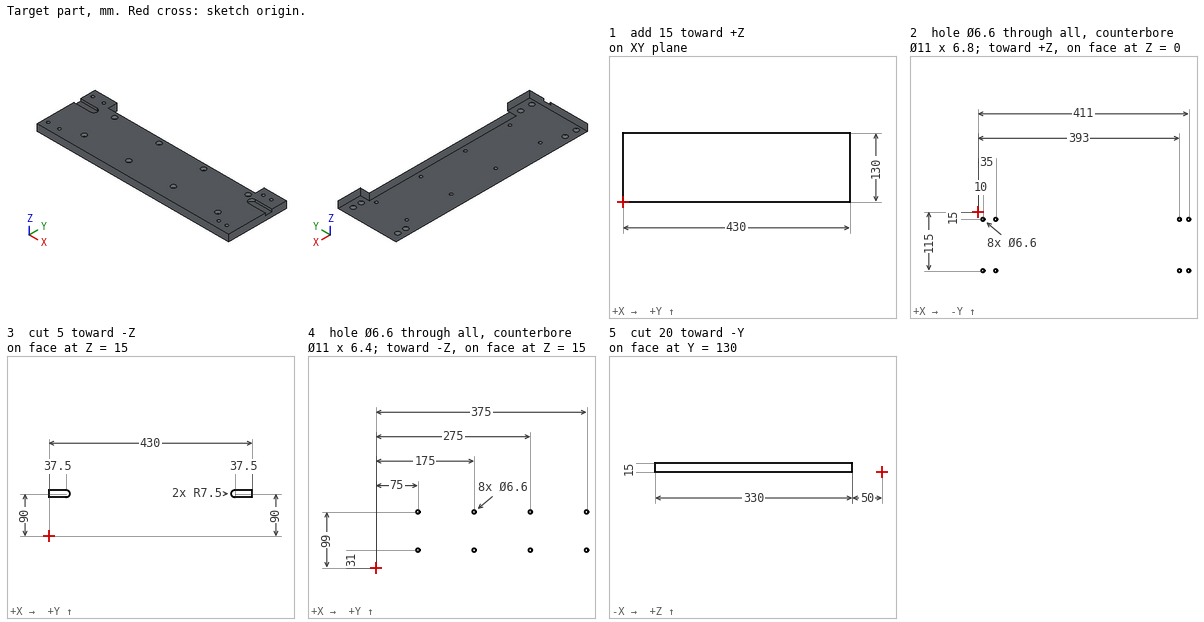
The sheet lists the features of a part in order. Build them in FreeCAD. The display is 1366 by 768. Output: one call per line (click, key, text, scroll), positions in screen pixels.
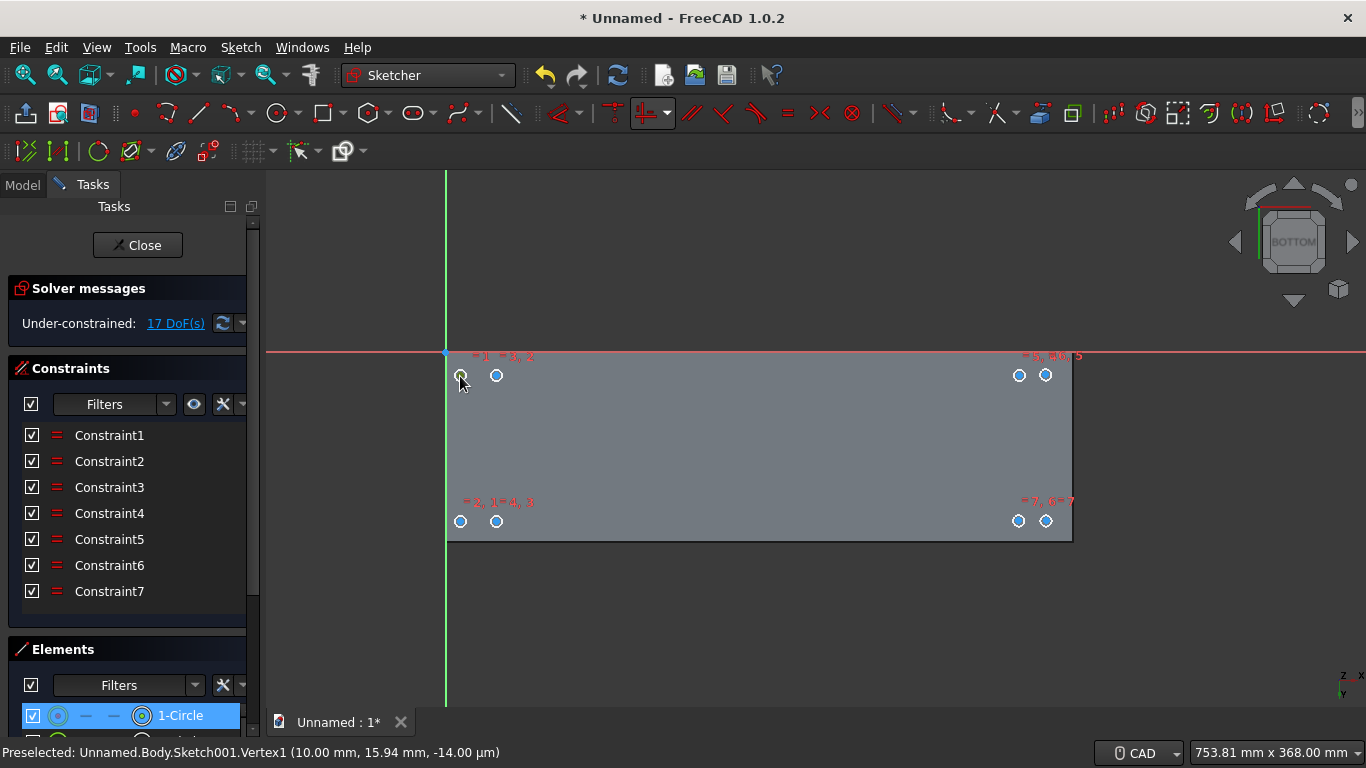
click(460, 522)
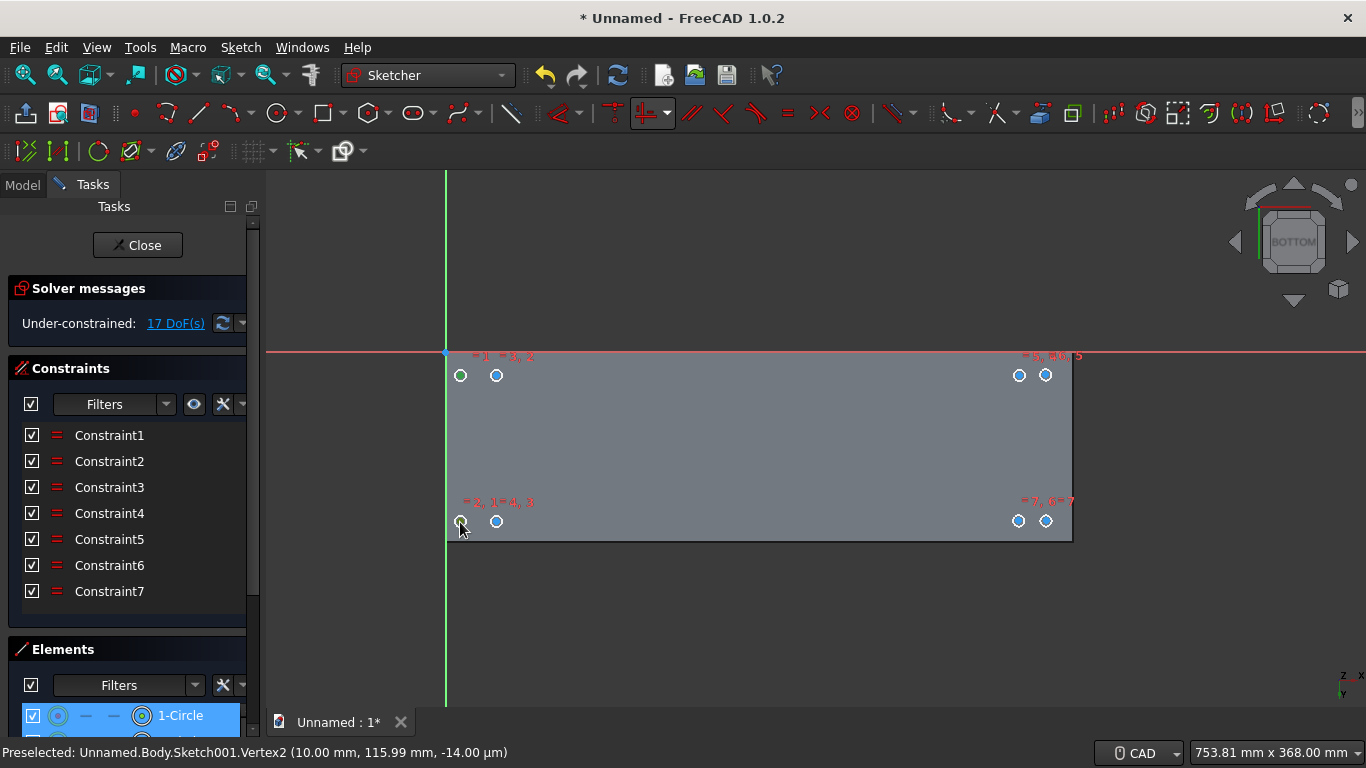
click(670, 114)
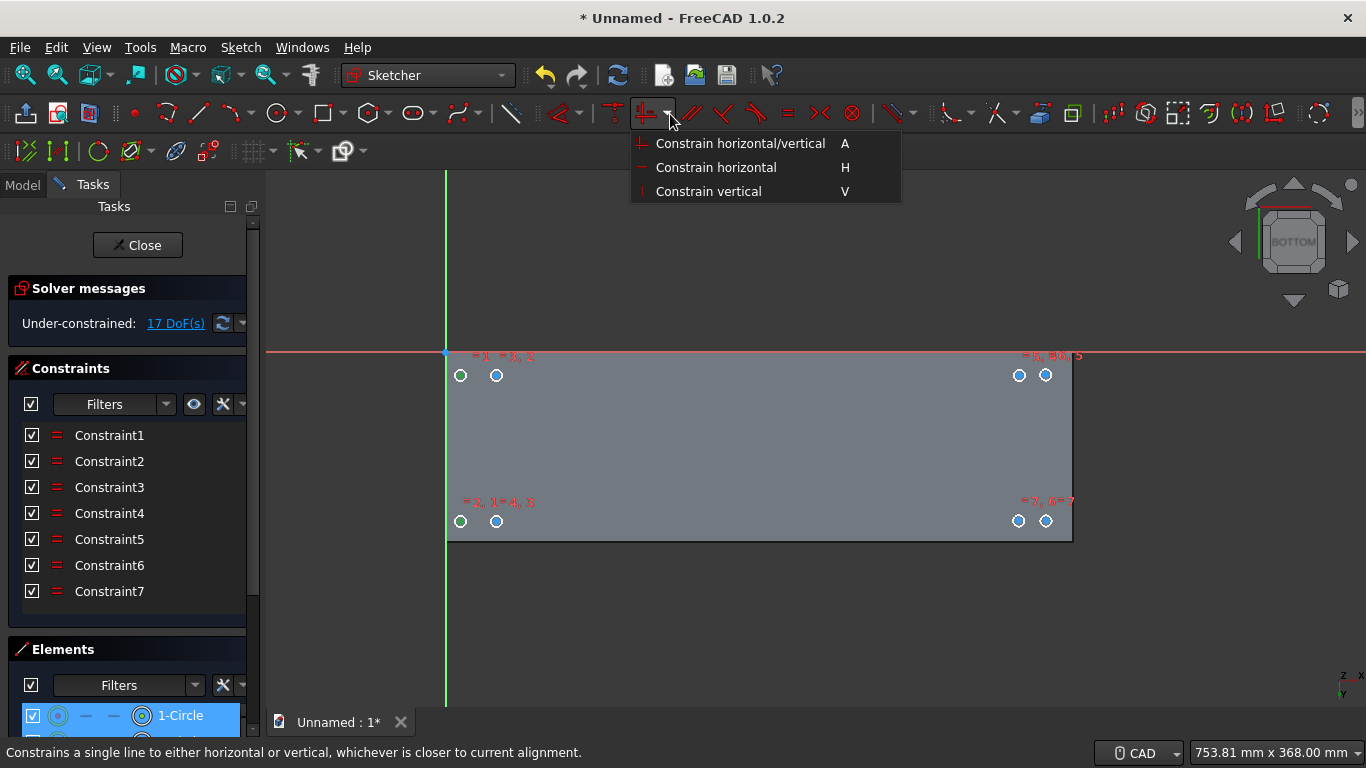
click(766, 191)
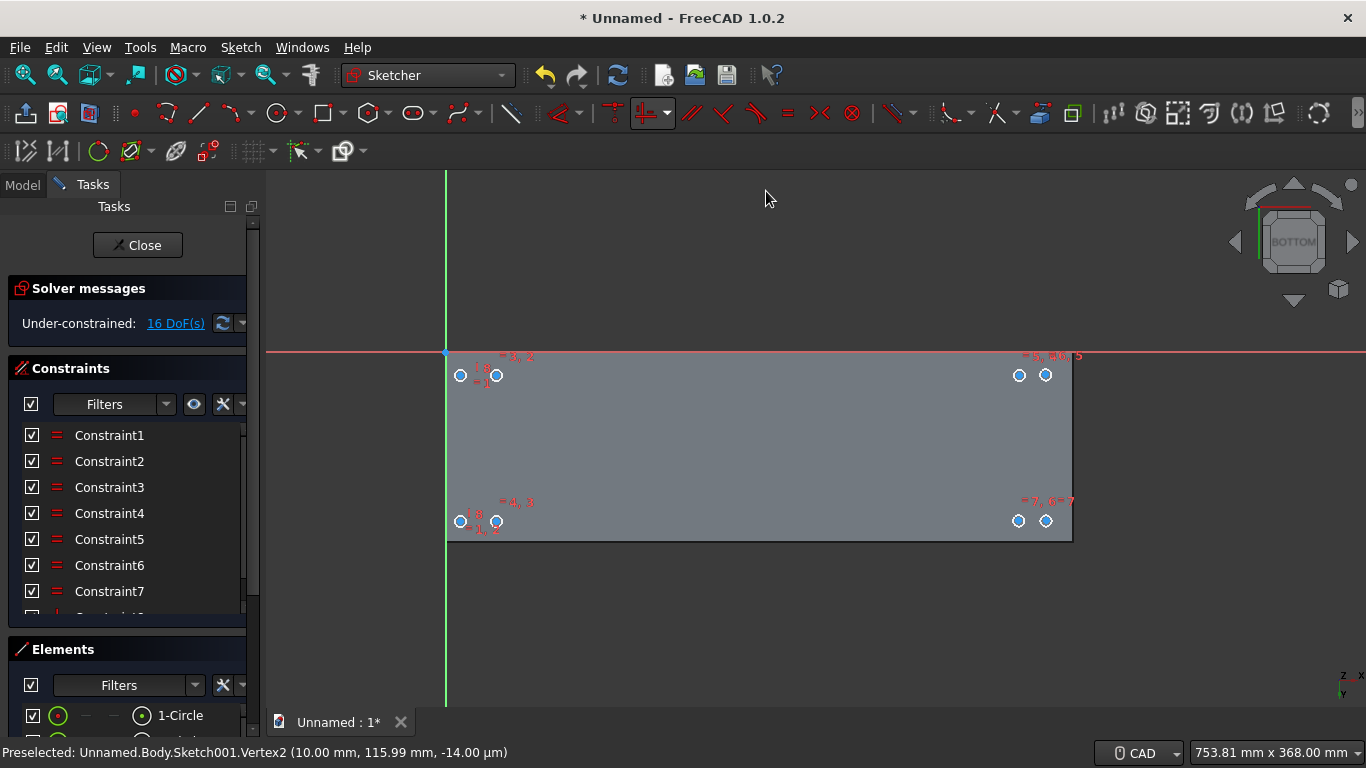
click(460, 376)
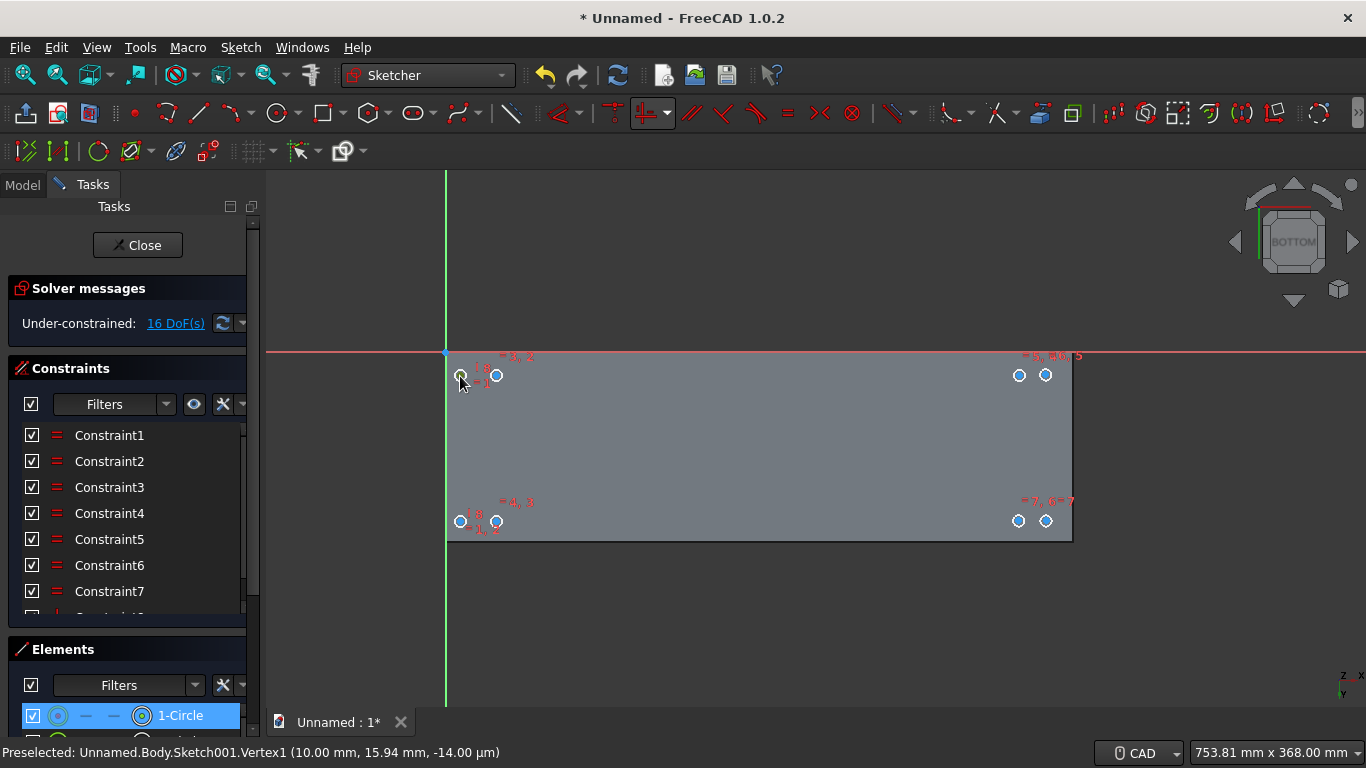
click(496, 376)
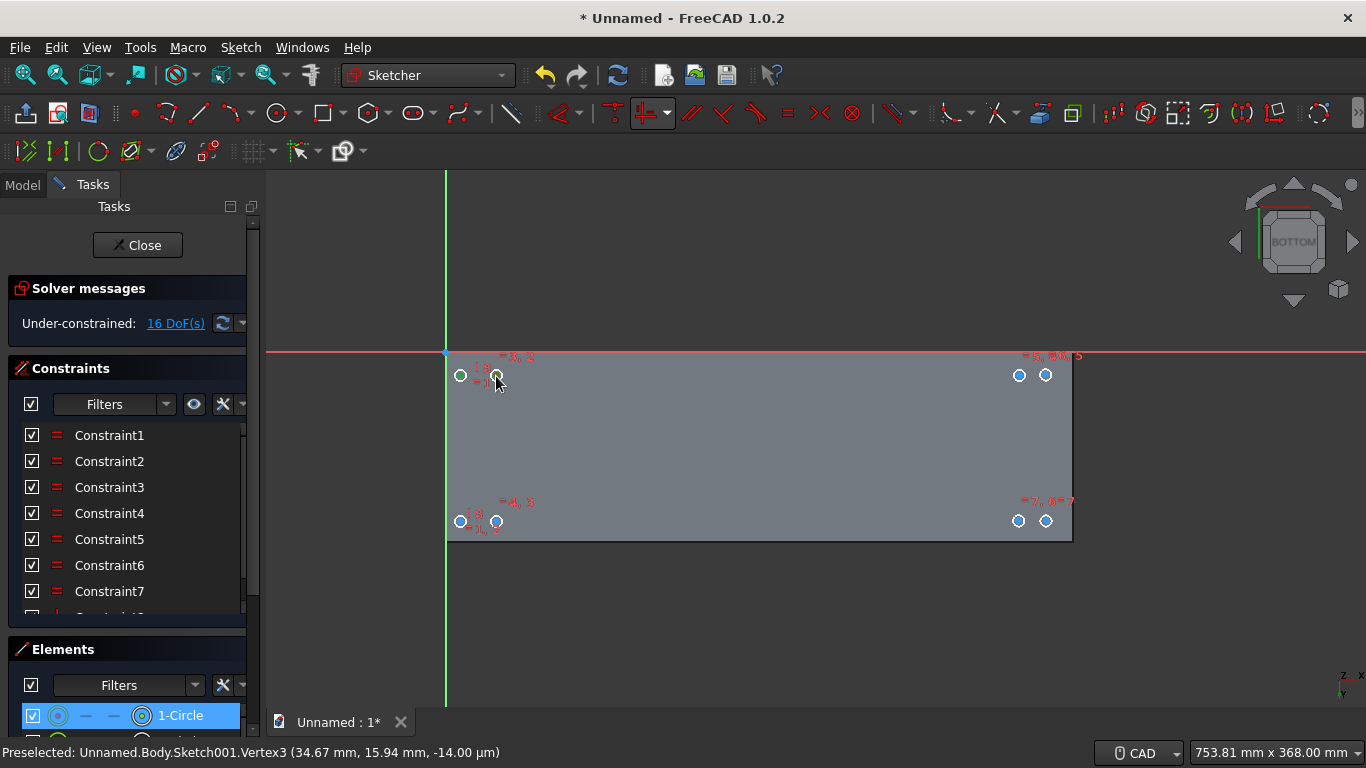
key(h)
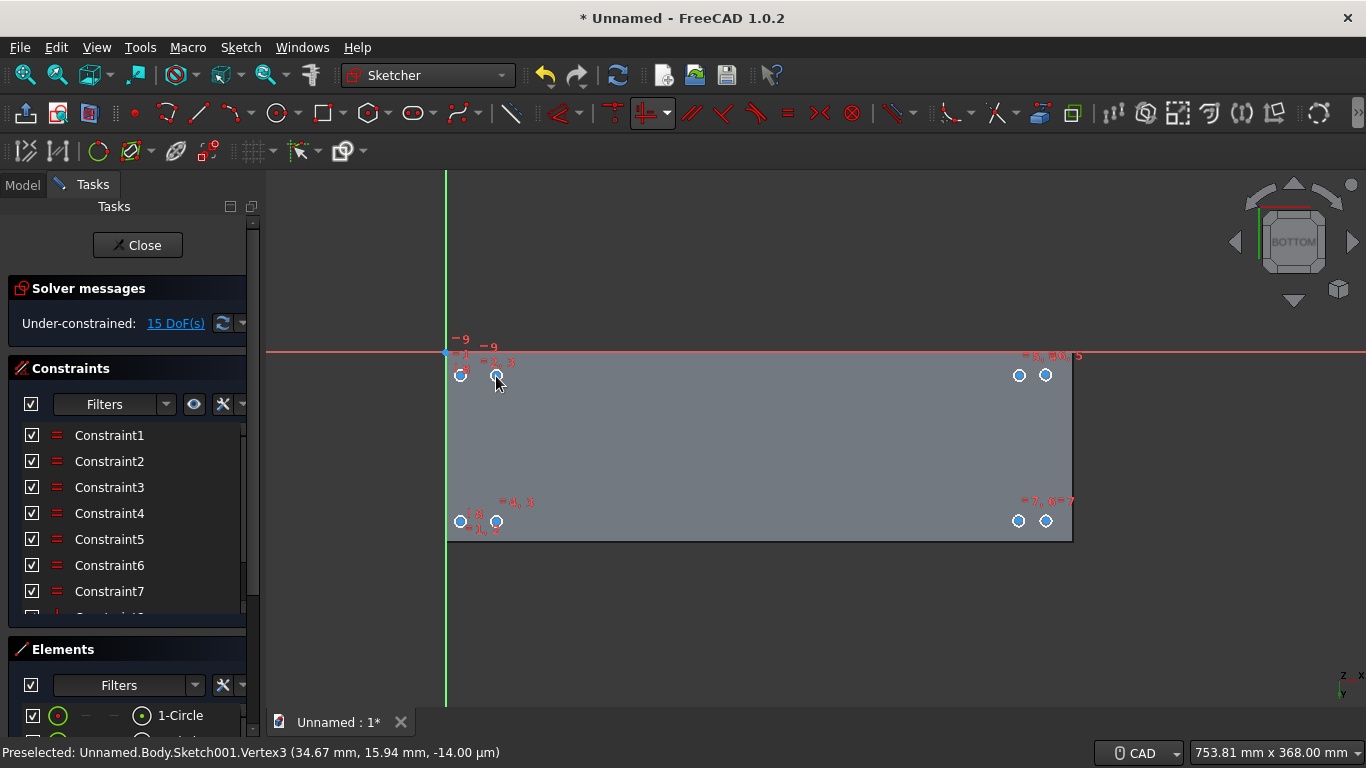
click(496, 376)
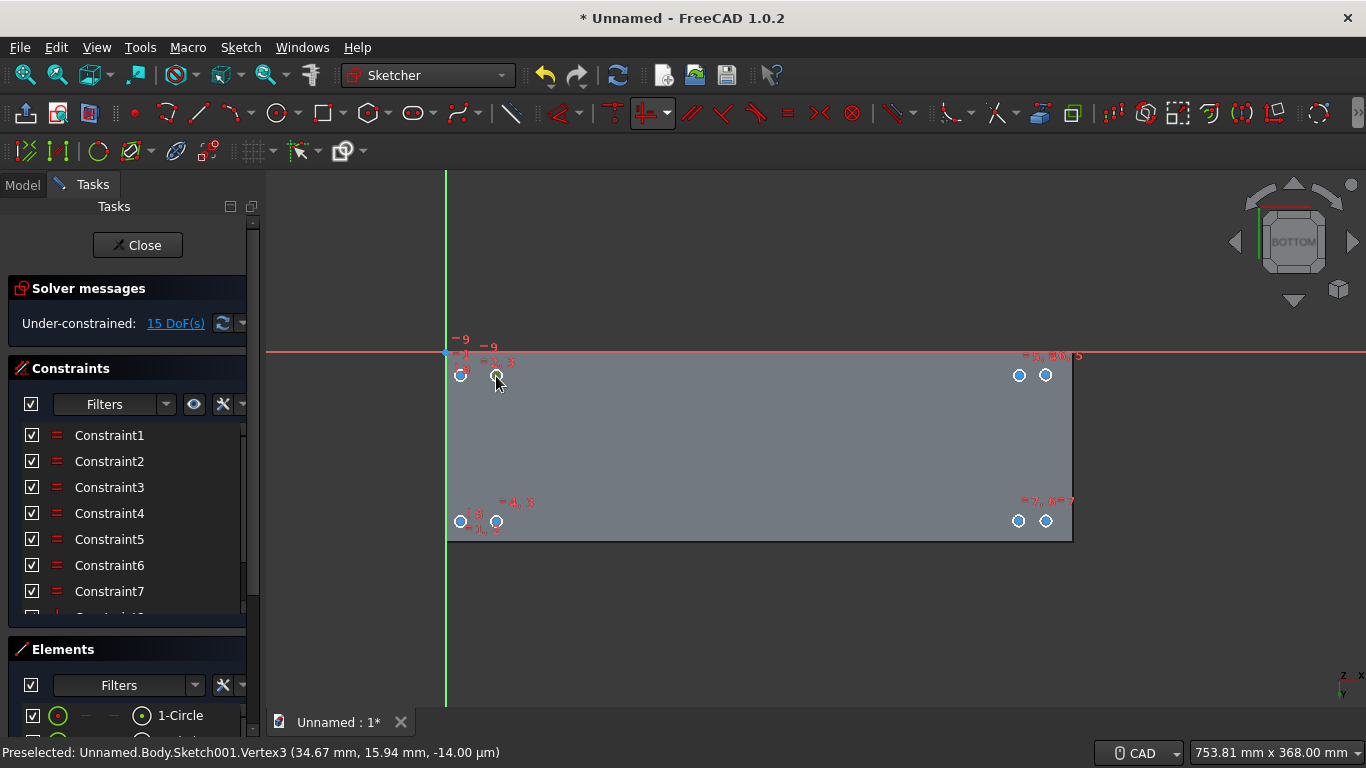
scroll(496, 522, up, 4)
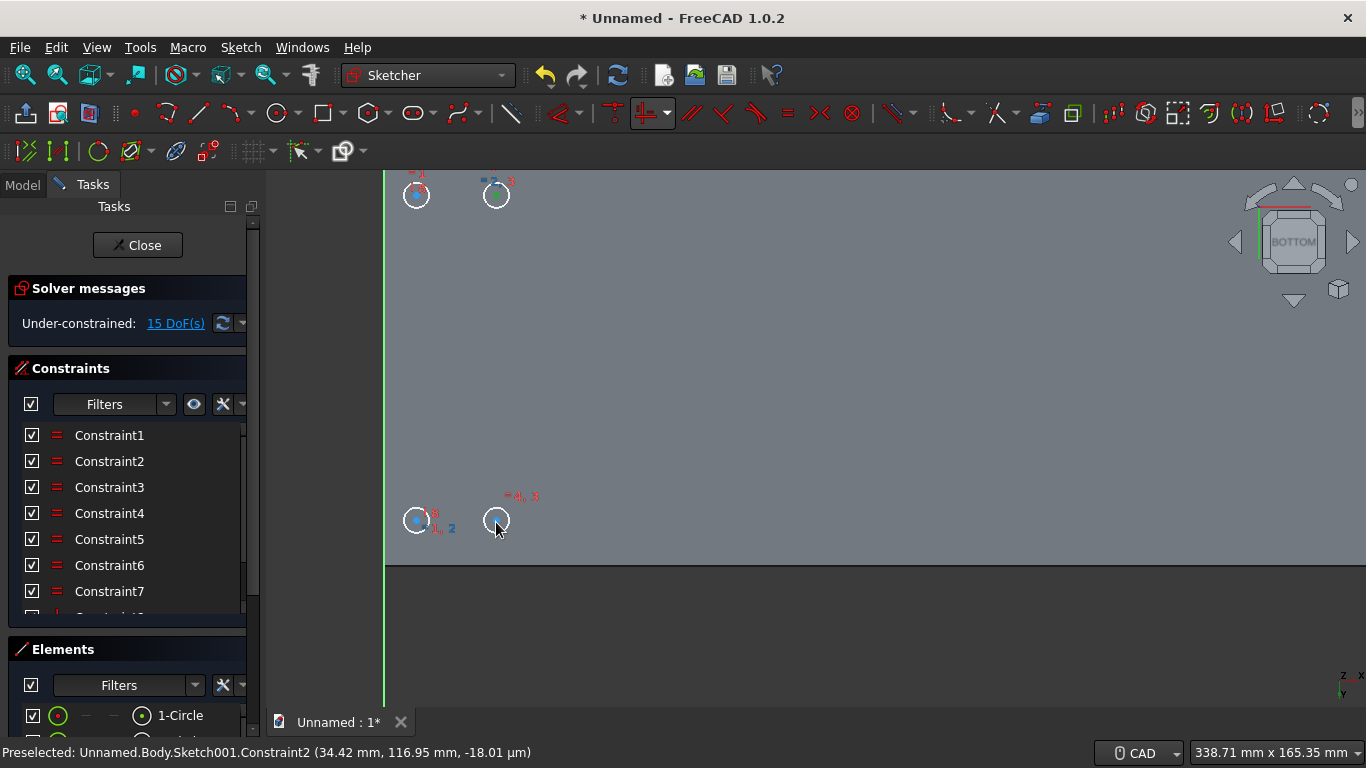
click(497, 520)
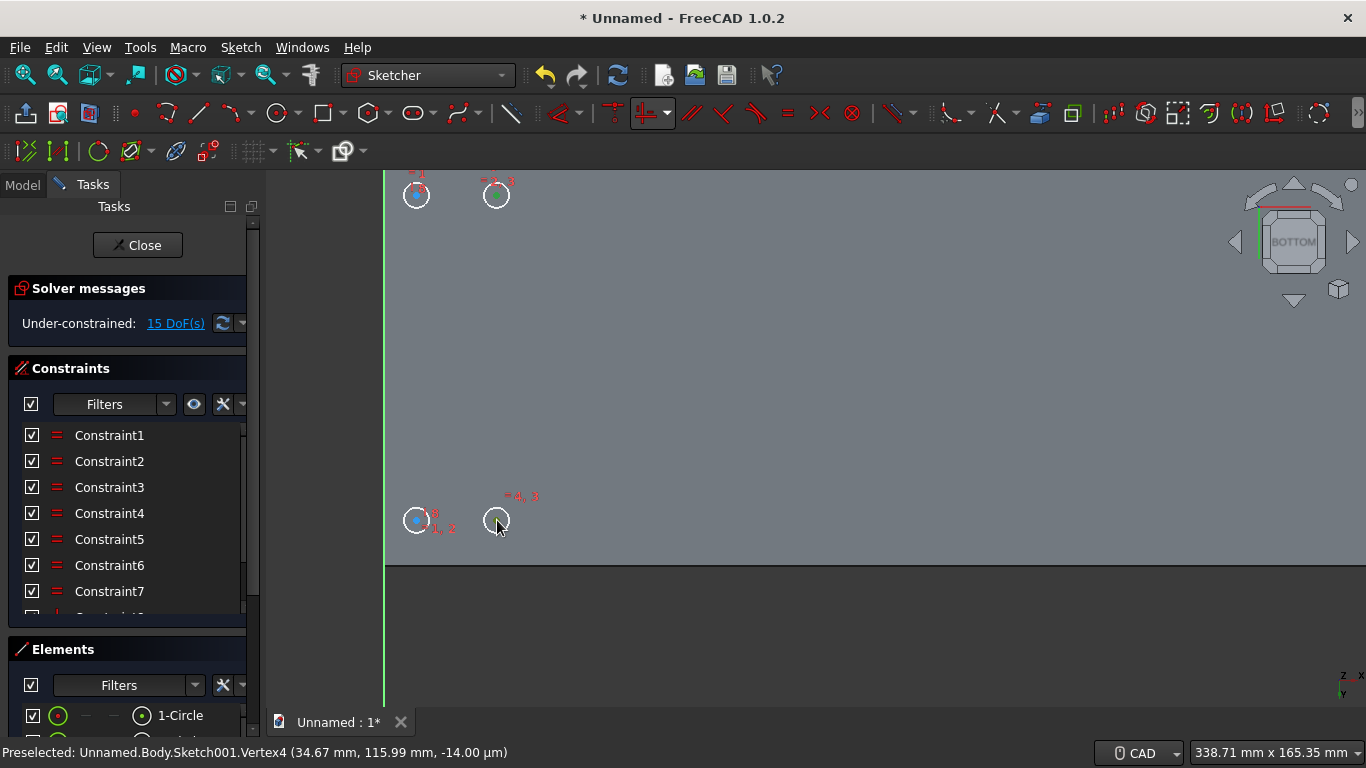
click(670, 114)